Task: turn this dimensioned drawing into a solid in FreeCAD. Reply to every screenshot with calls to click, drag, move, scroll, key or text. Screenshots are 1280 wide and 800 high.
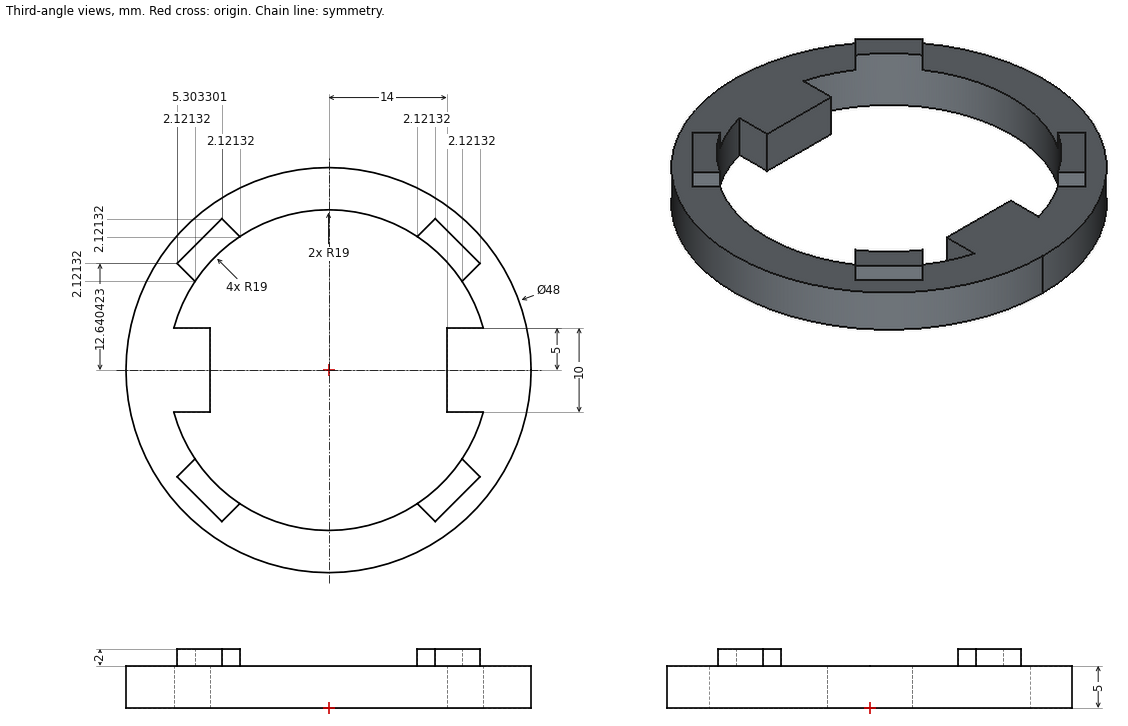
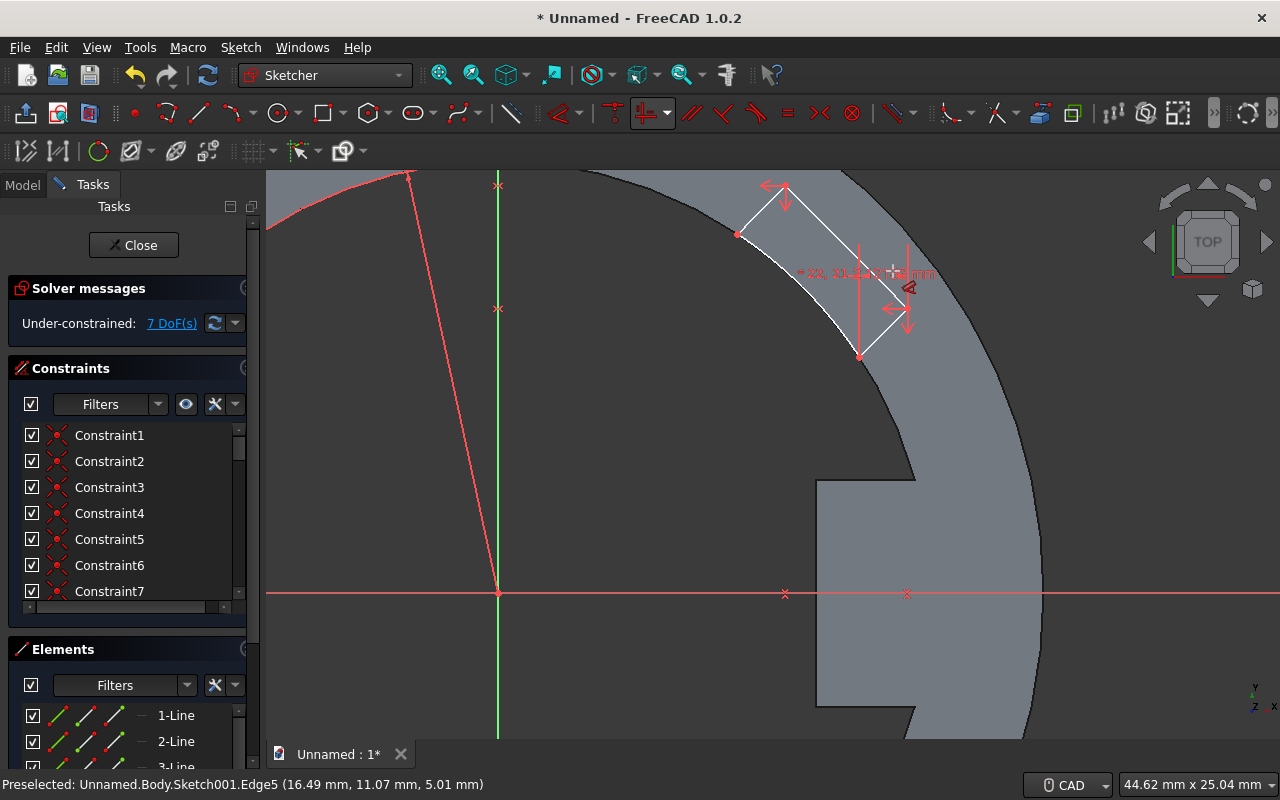
click(771, 200)
click(762, 268)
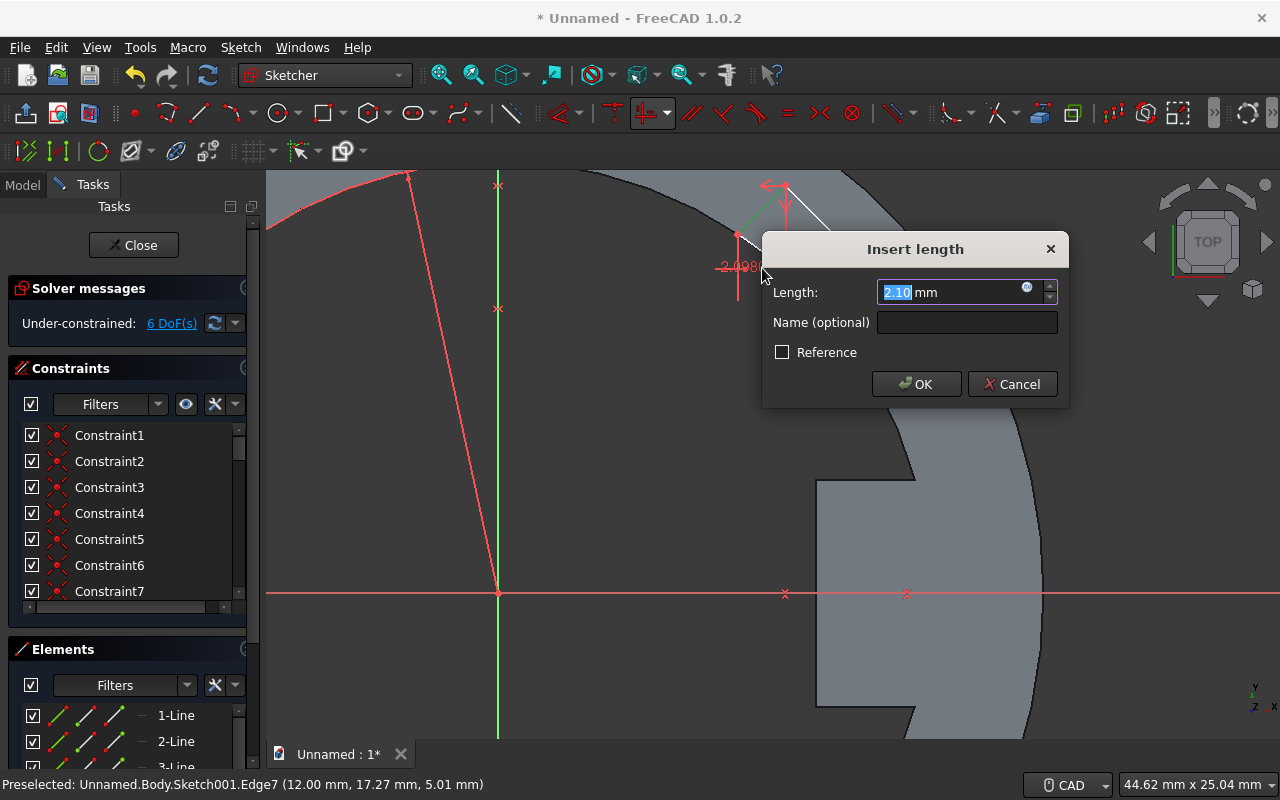
text(2.12132)
key(Return)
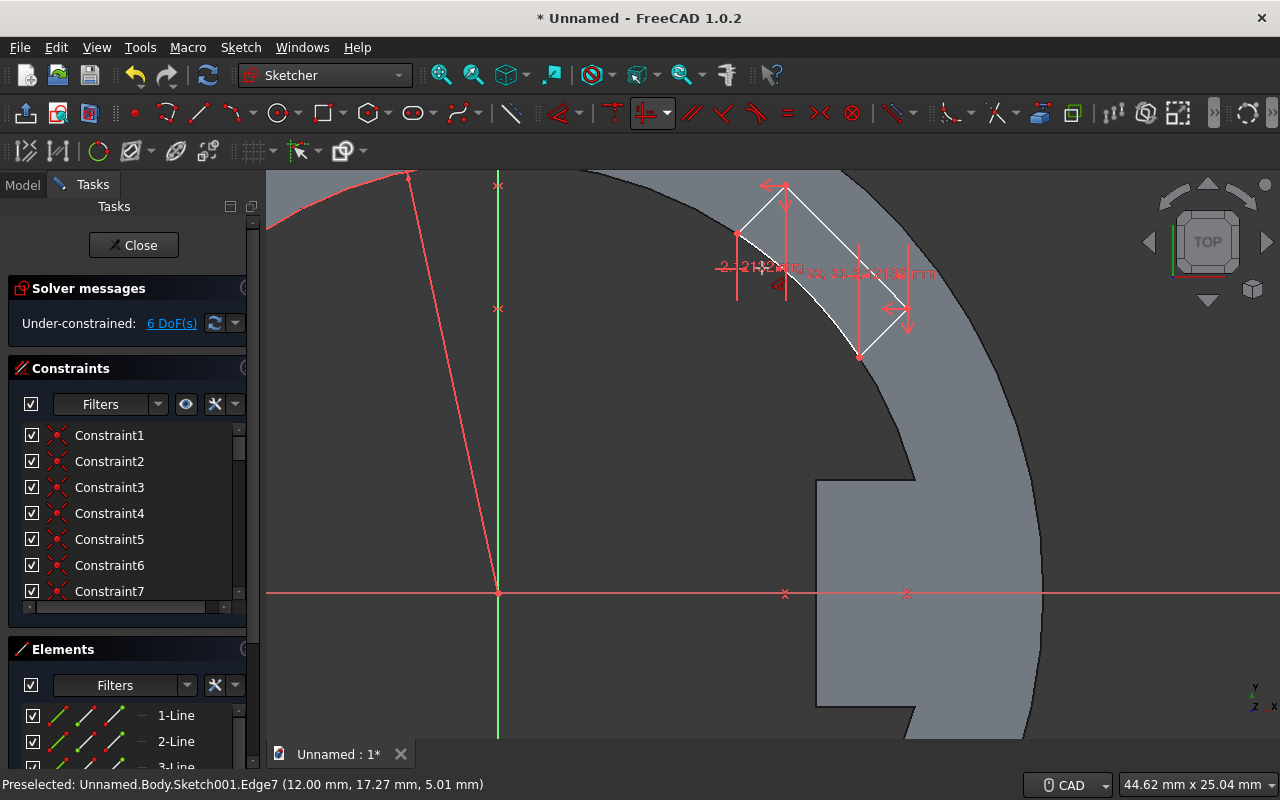
scroll(873, 341, down, 4)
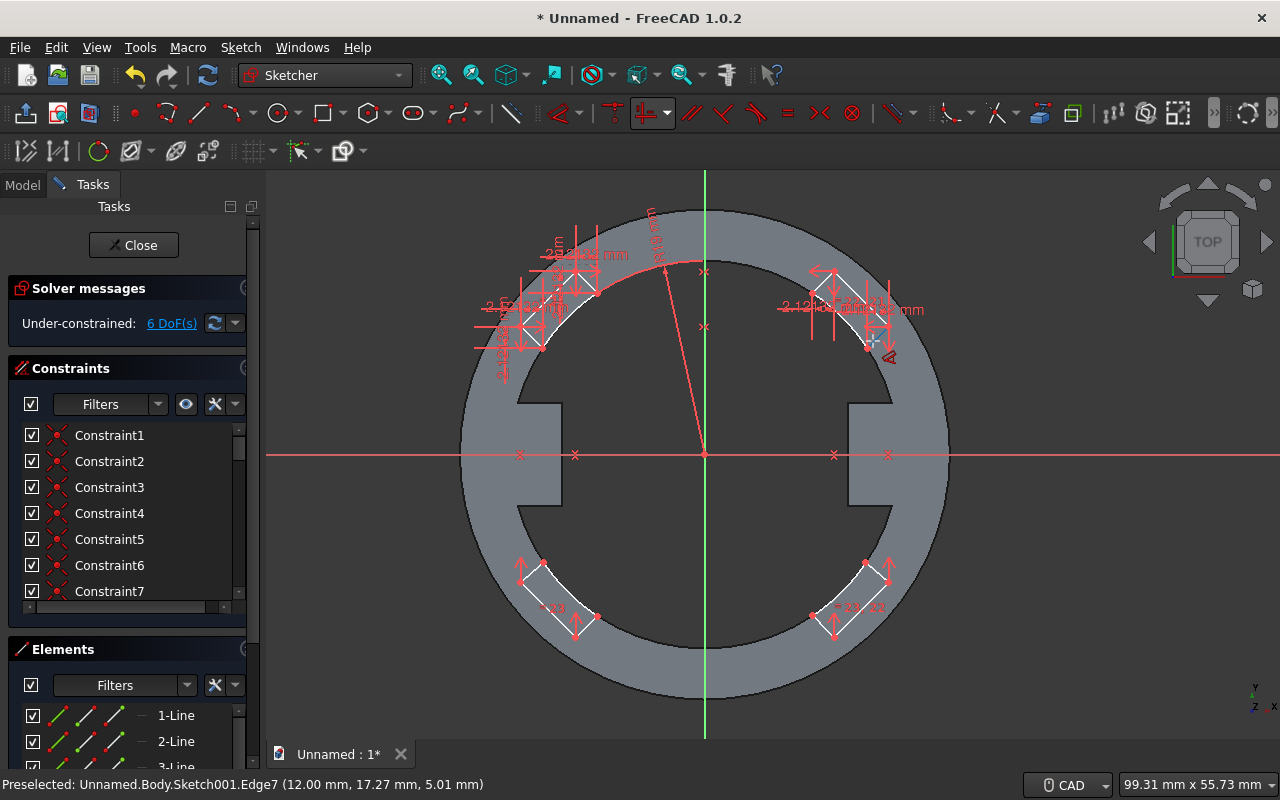
scroll(819, 622, up, 4)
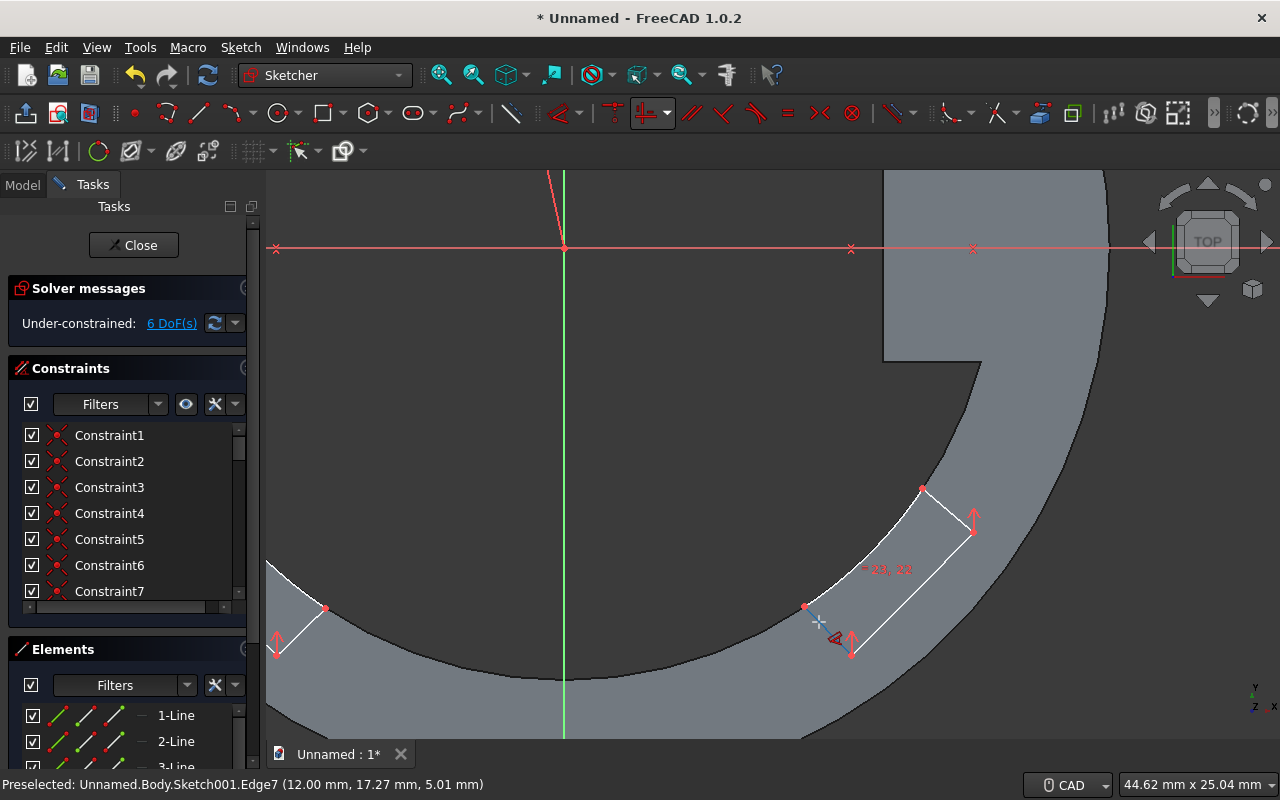
click(819, 622)
click(828, 690)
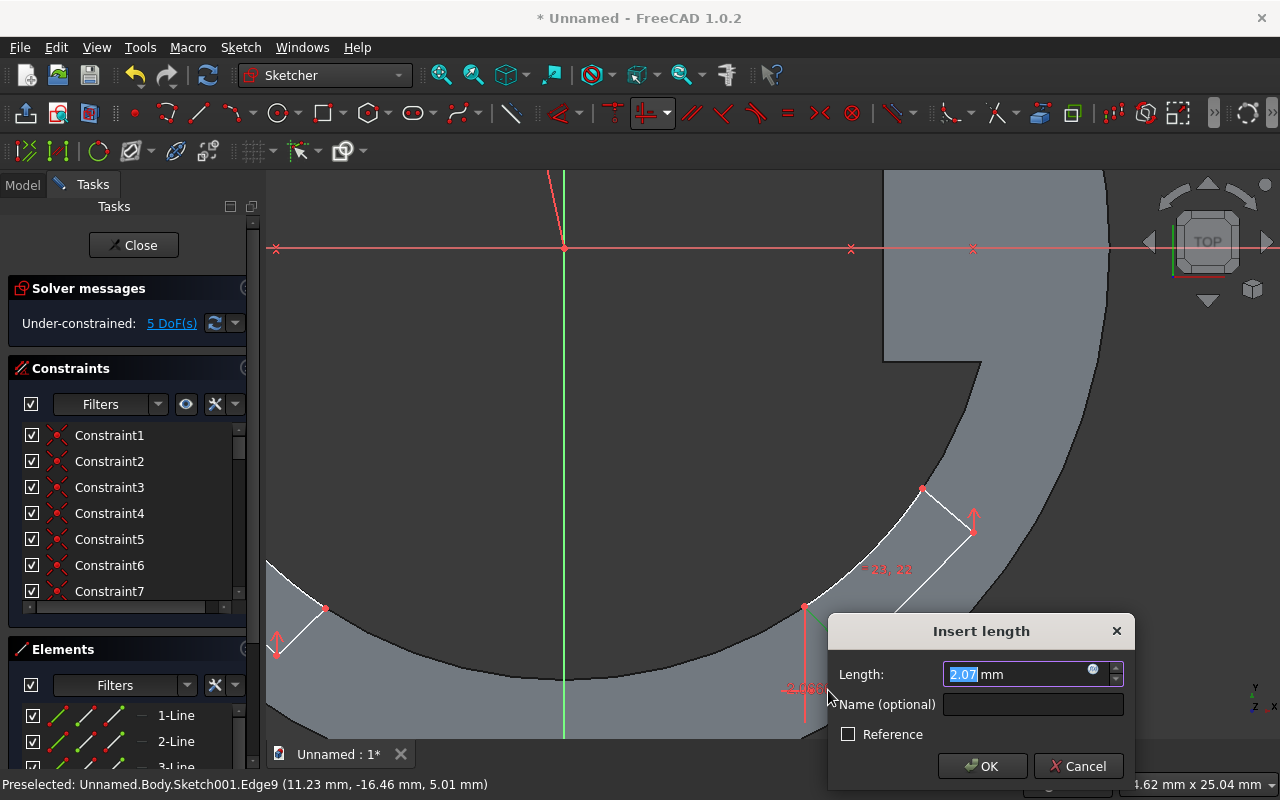
text(2.12132)
key(Return)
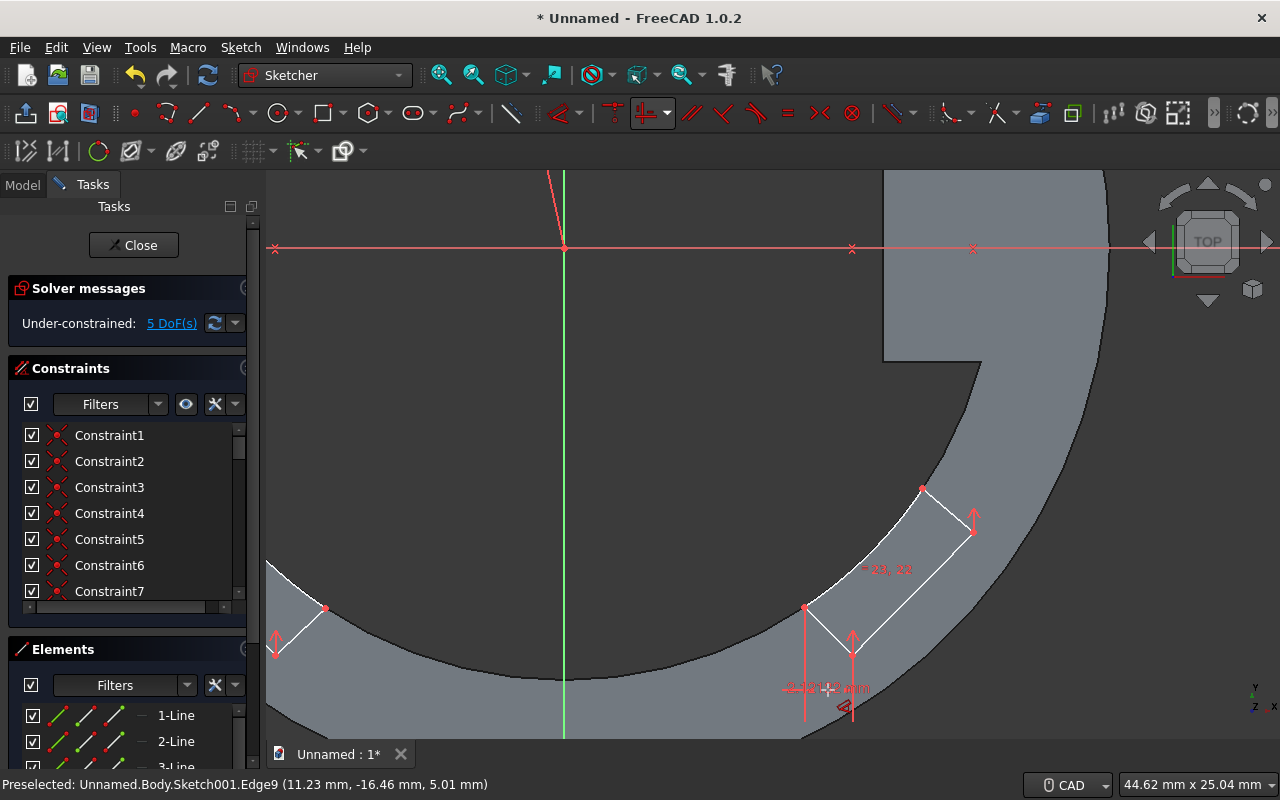
click(959, 520)
click(960, 567)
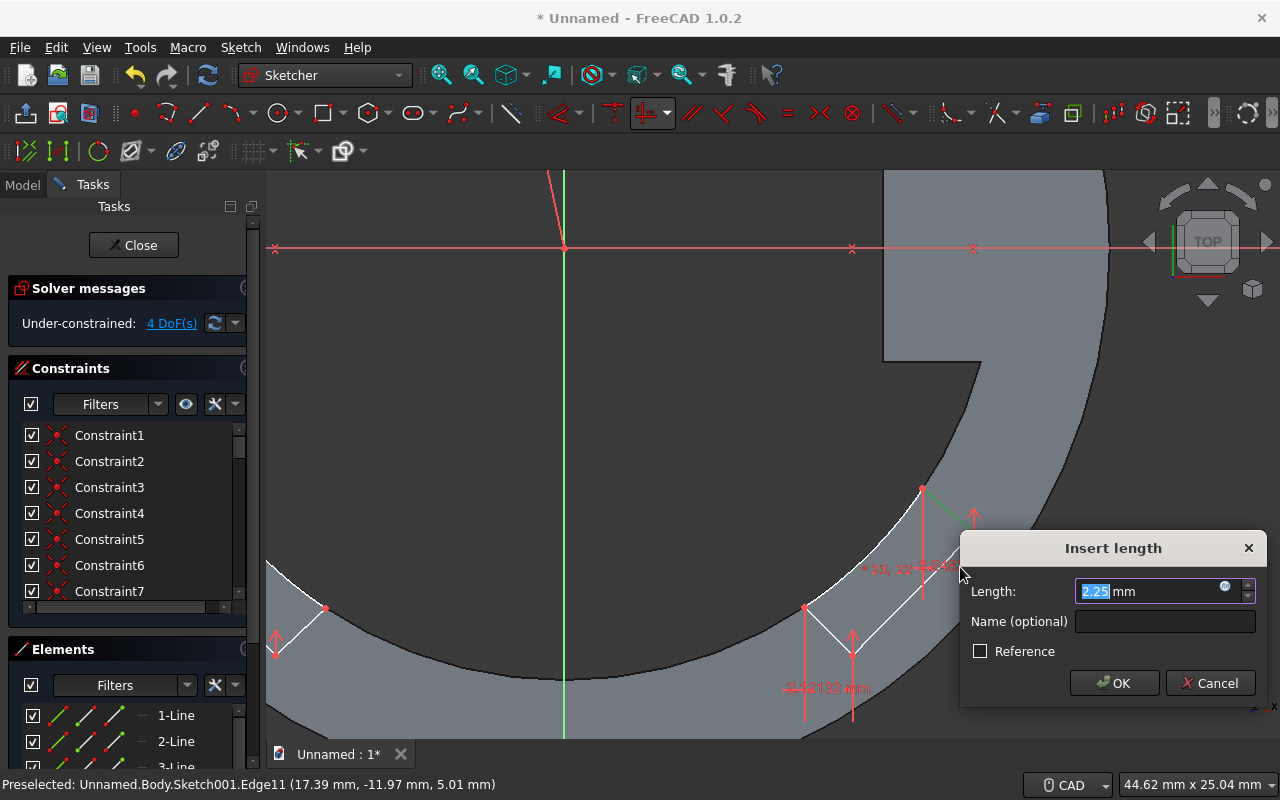
text(2.12132)
key(Return)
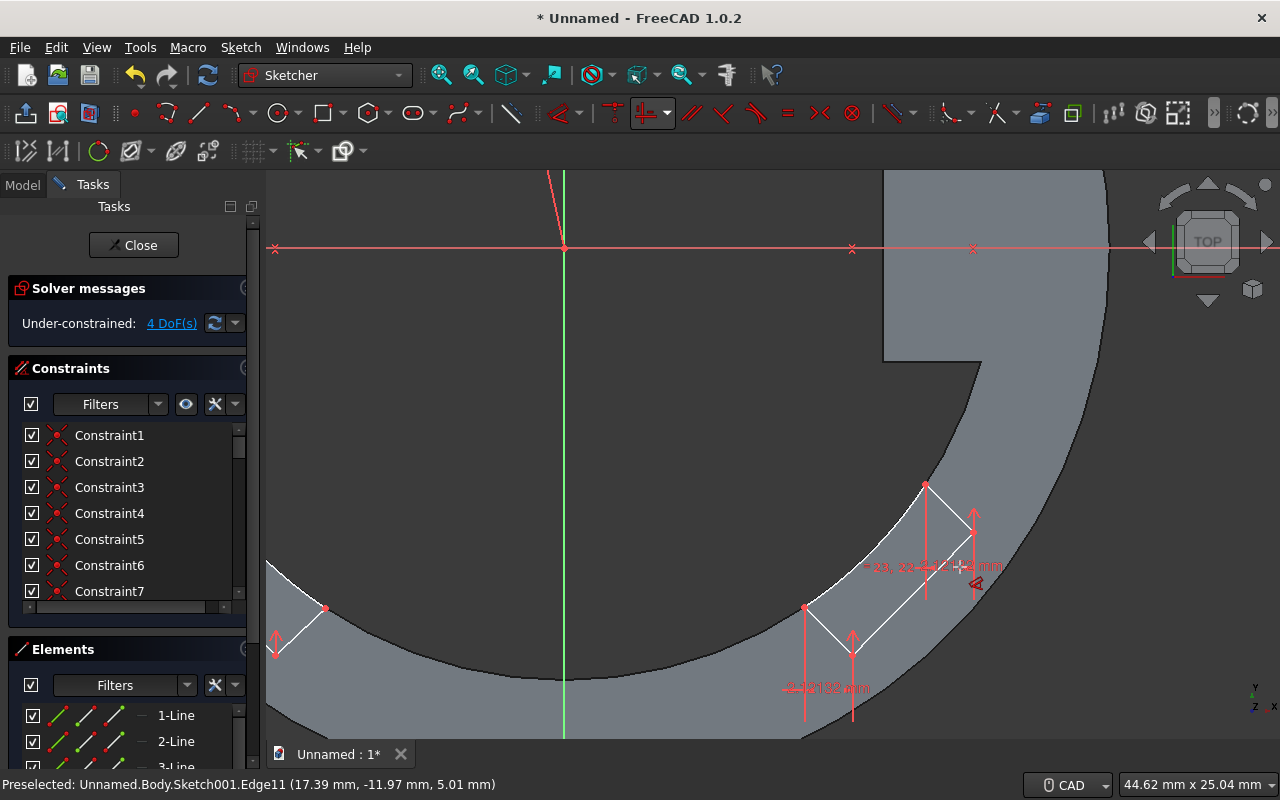
scroll(819, 623, down, 4)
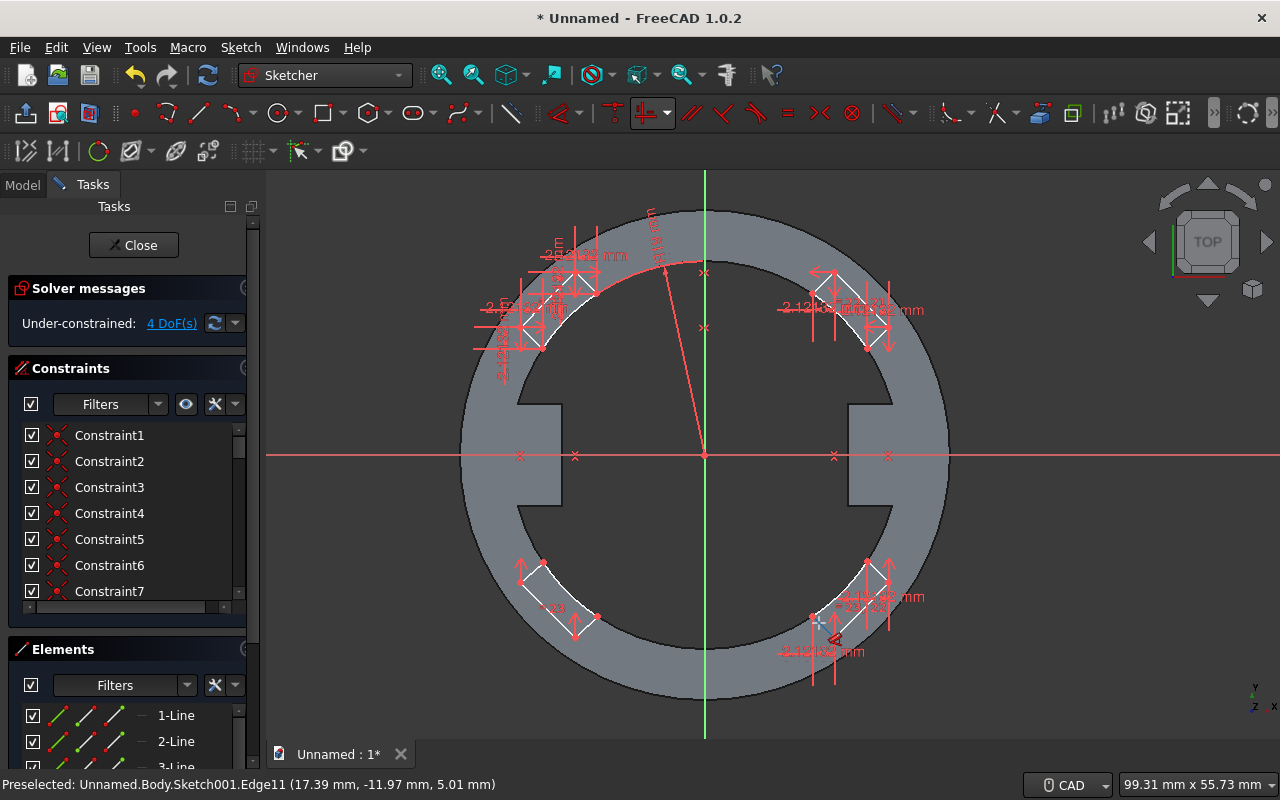
scroll(537, 569, up, 4)